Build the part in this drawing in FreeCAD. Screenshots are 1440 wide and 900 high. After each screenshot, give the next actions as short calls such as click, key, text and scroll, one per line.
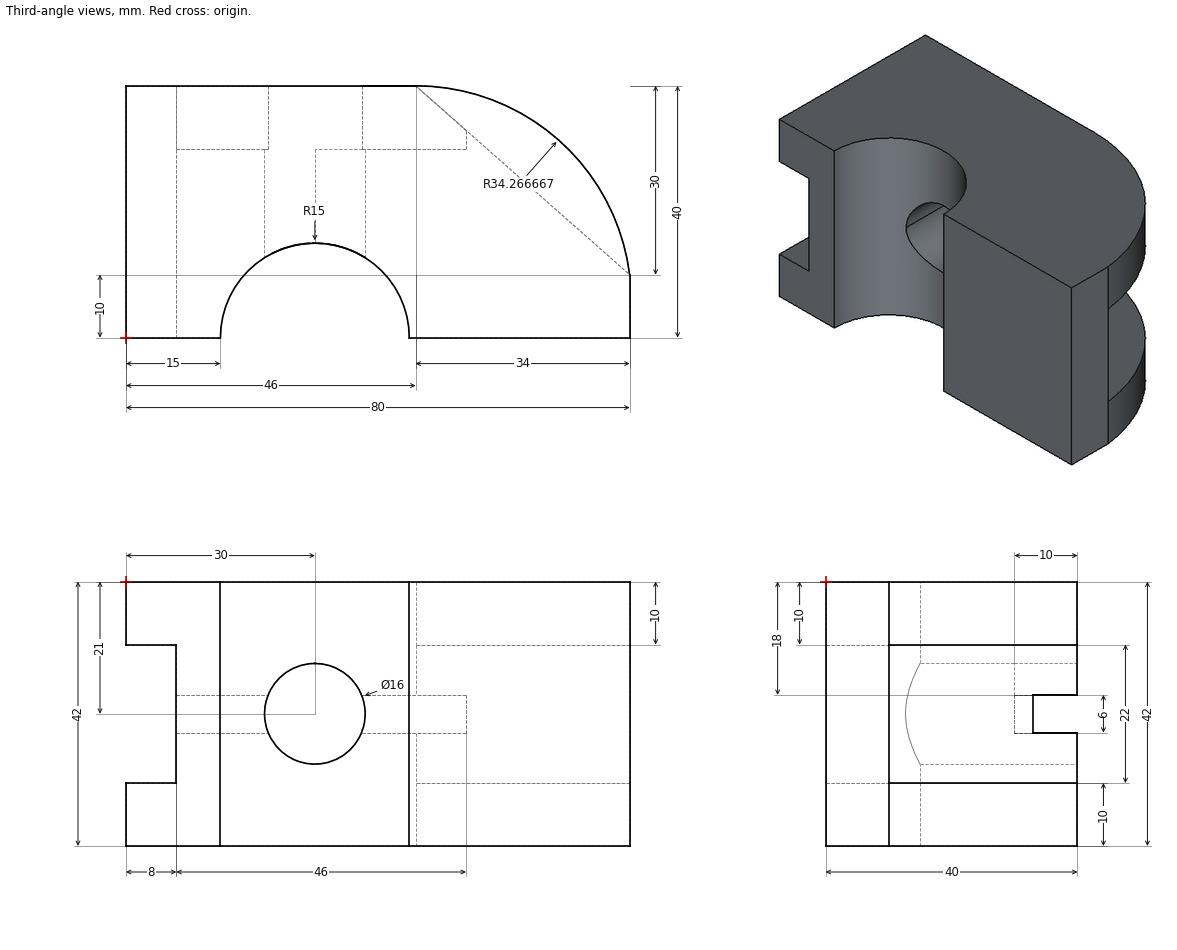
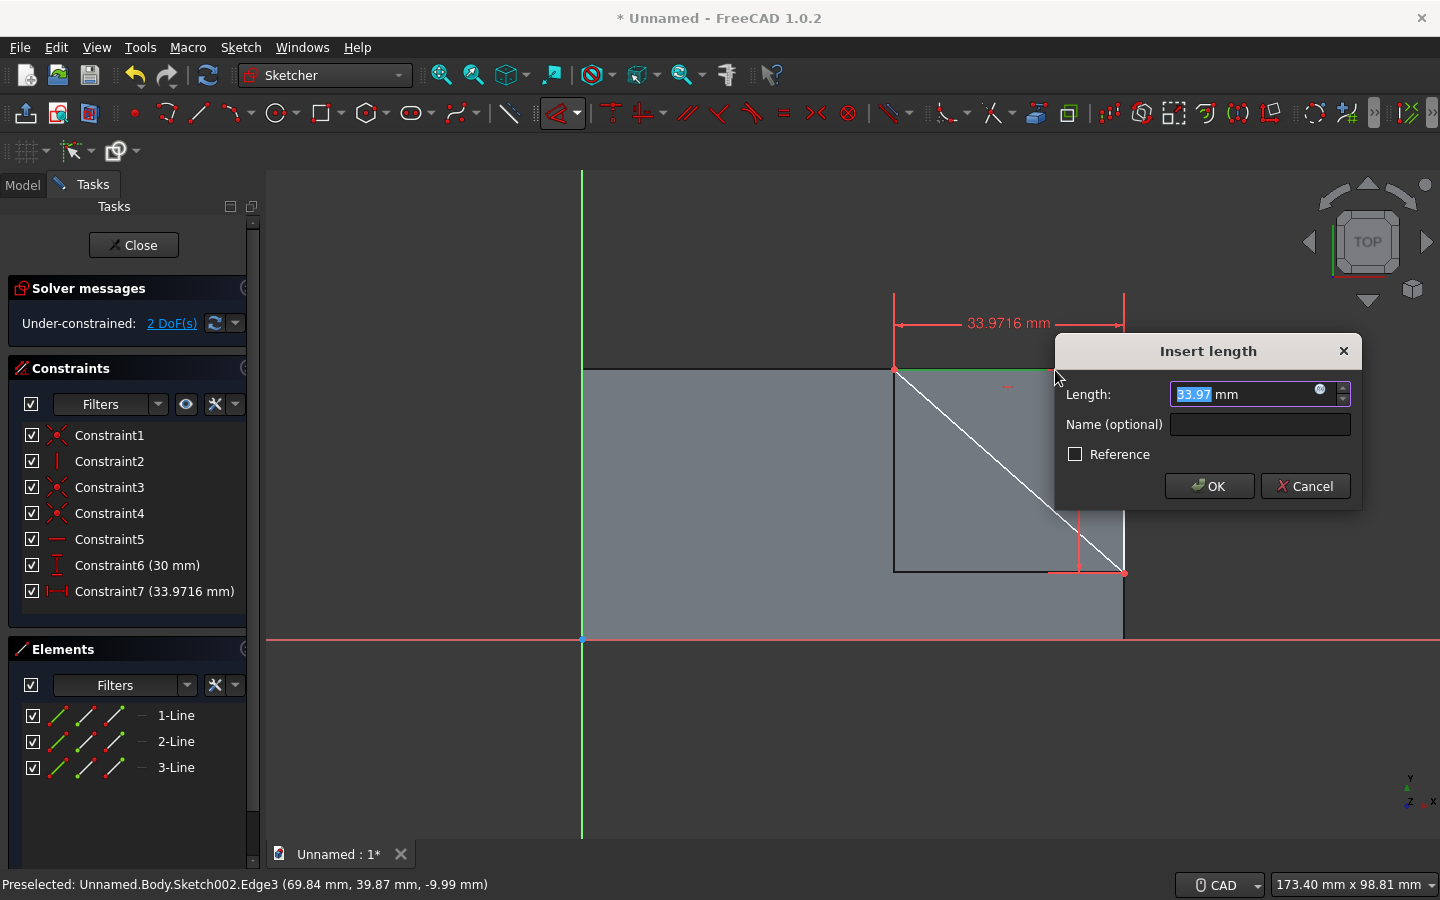
text(34)
key(Return)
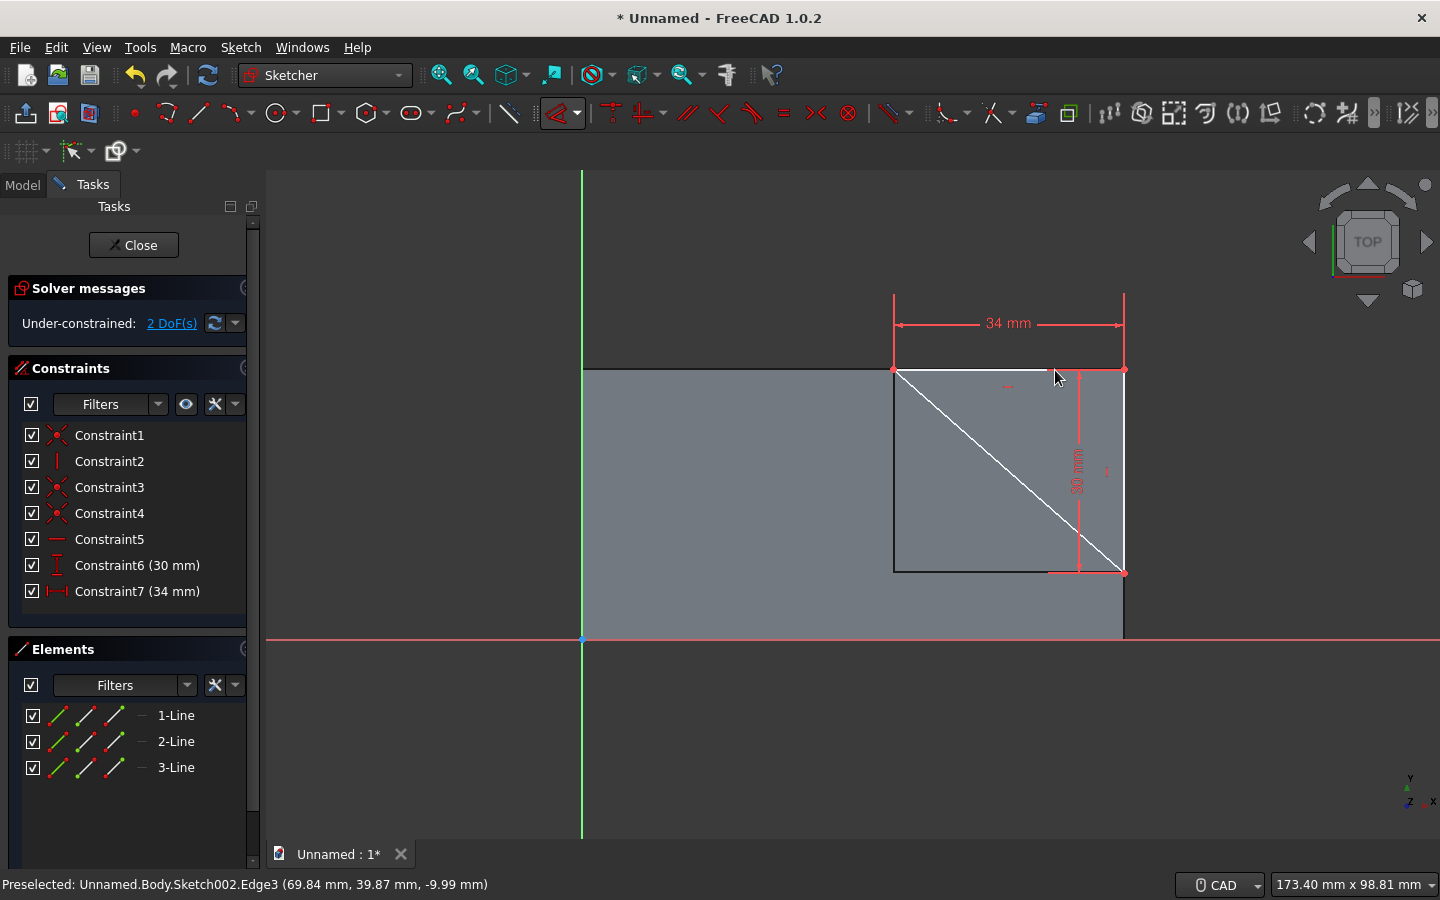
click(894, 370)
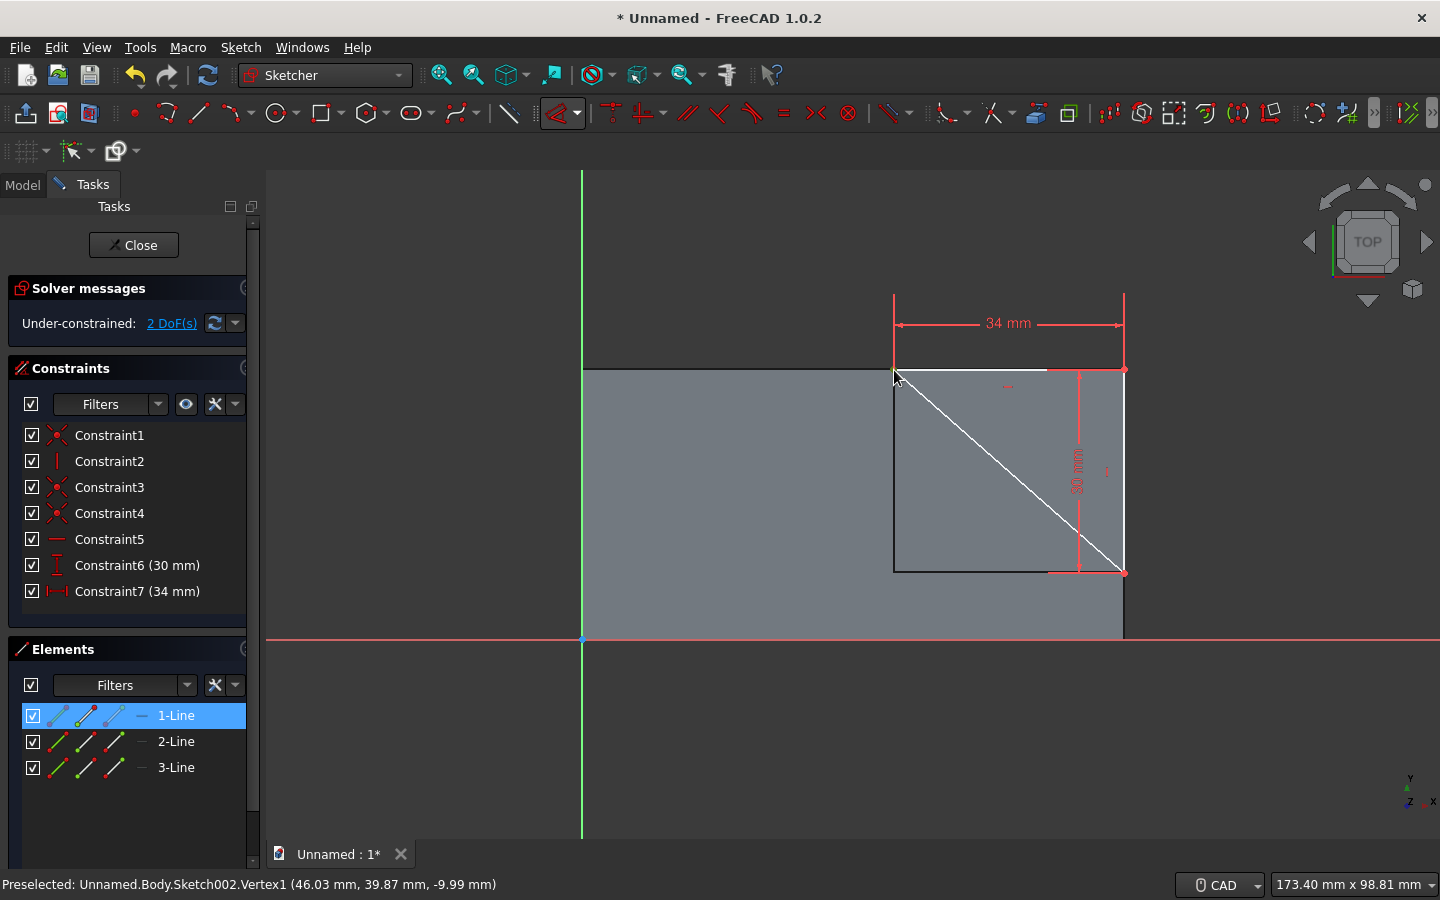
click(580, 114)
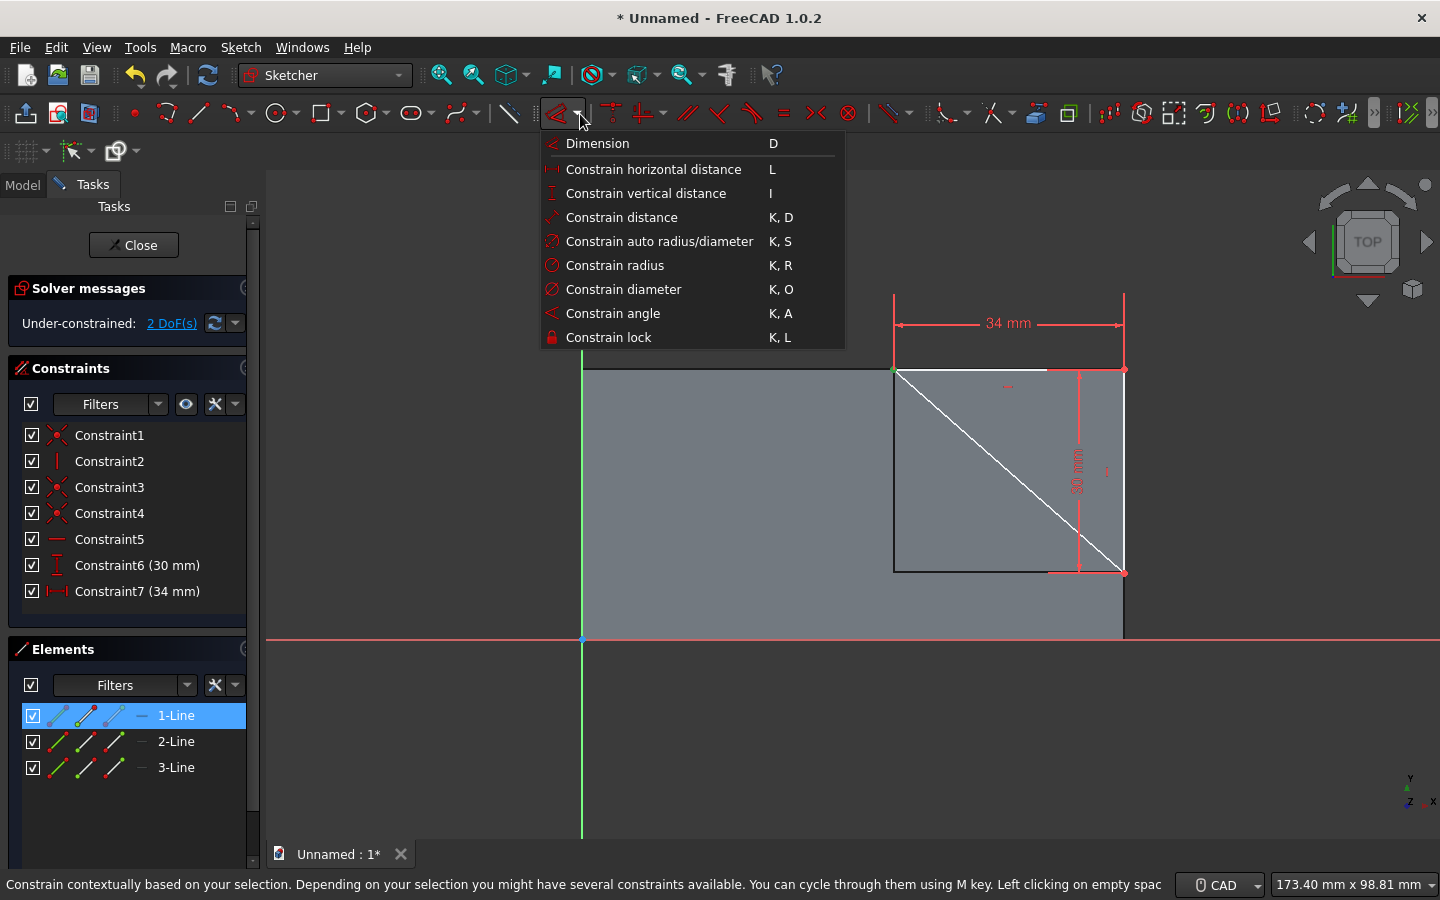
click(693, 169)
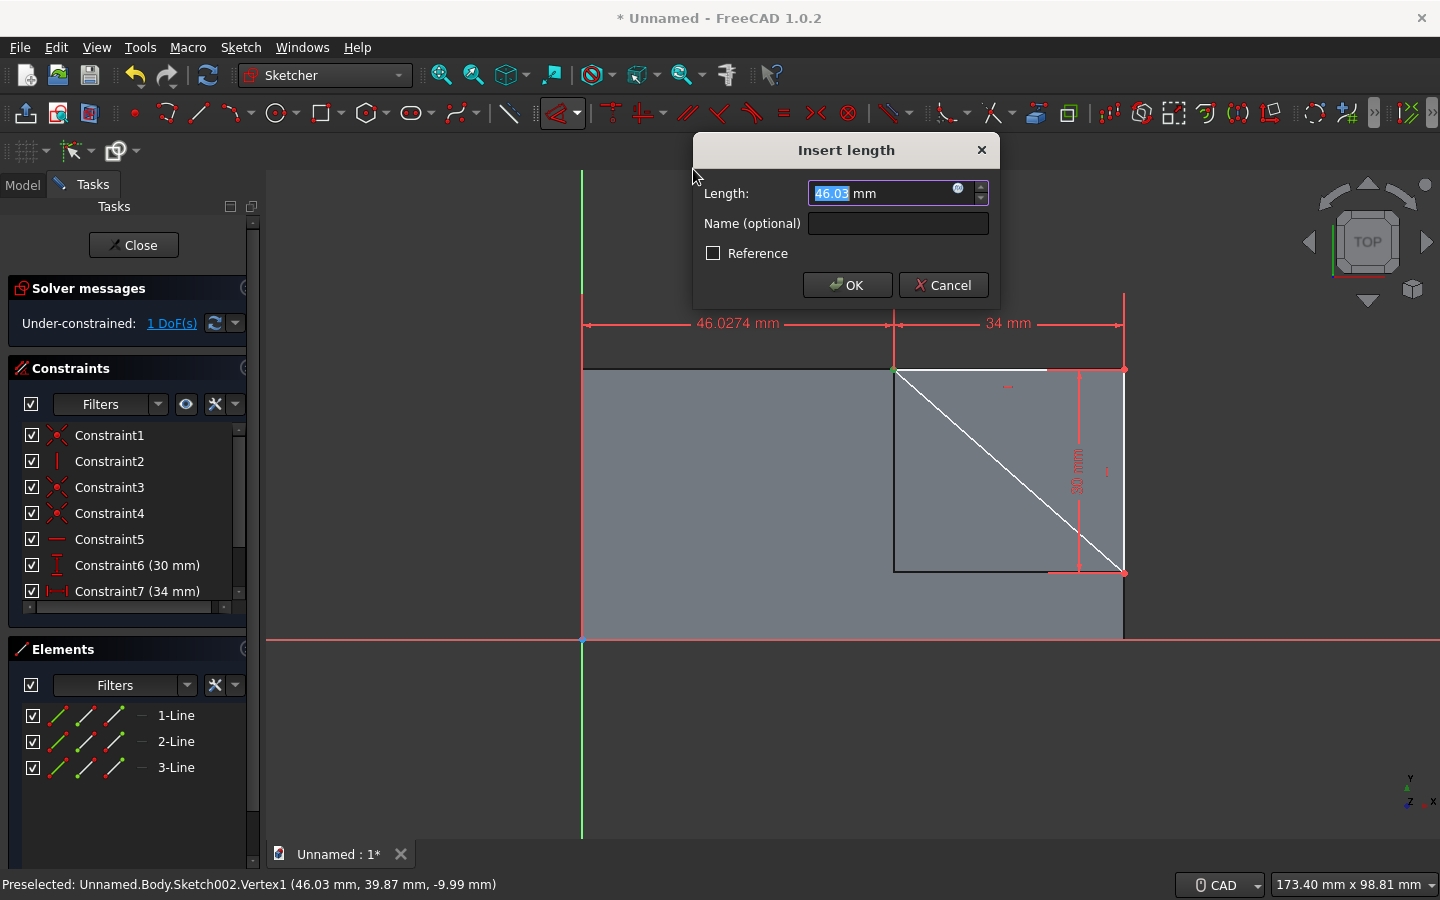
text(46)
key(Return)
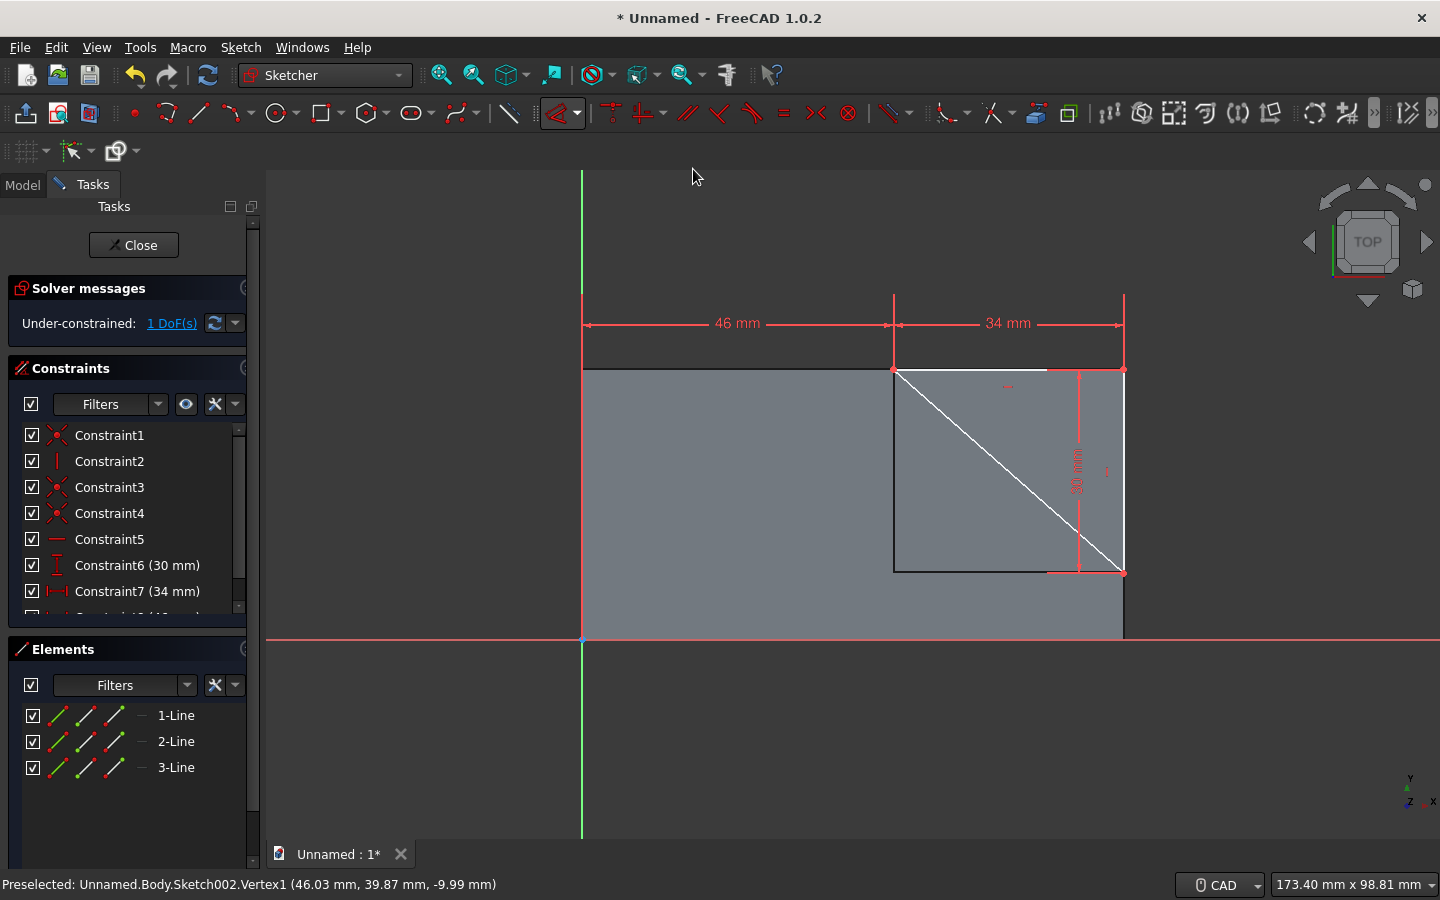
click(894, 370)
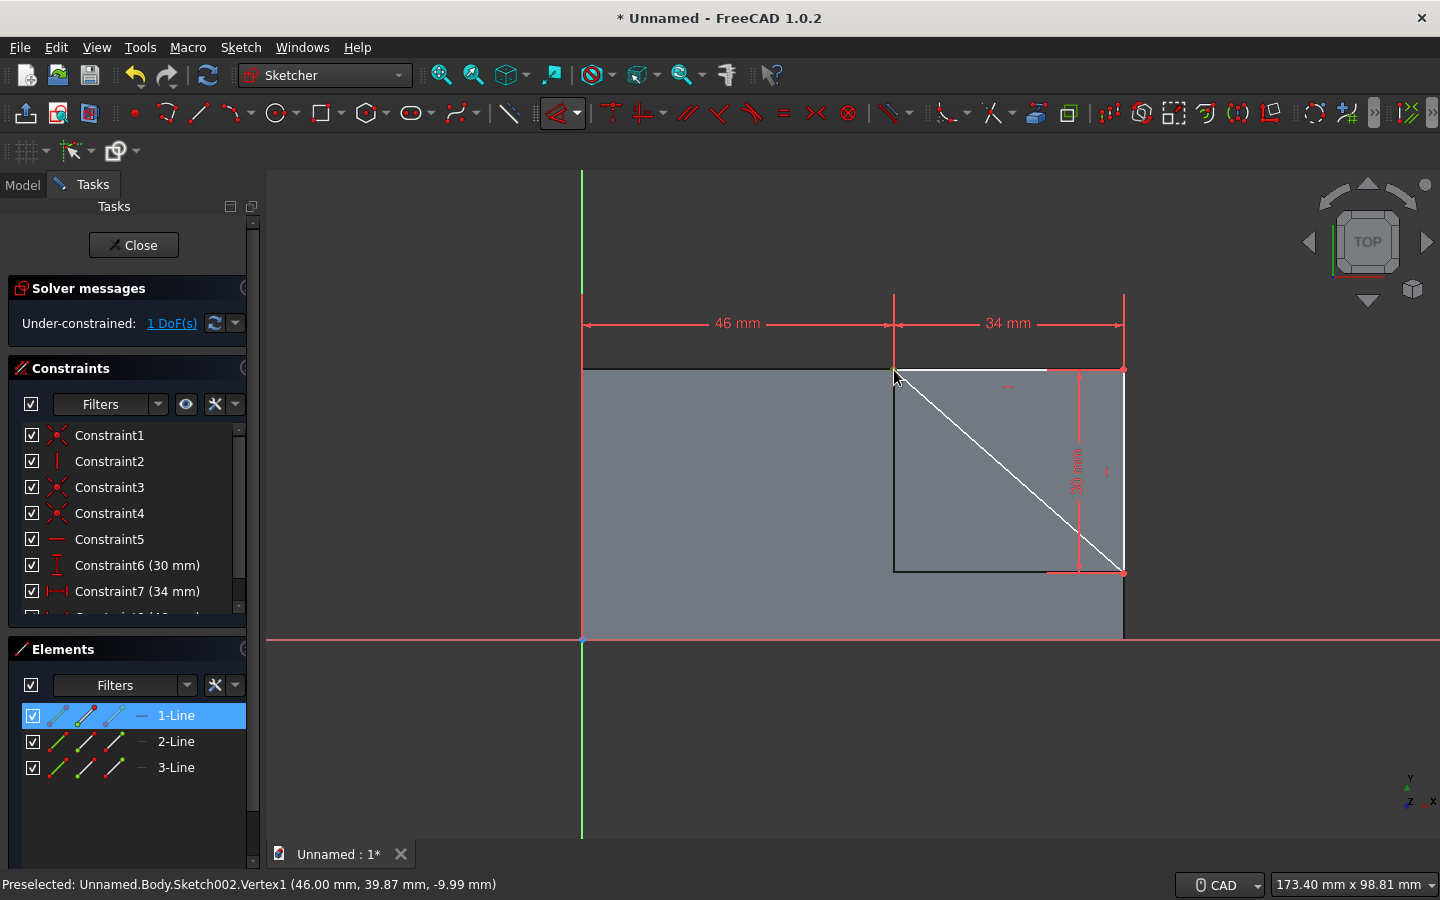
key(i)